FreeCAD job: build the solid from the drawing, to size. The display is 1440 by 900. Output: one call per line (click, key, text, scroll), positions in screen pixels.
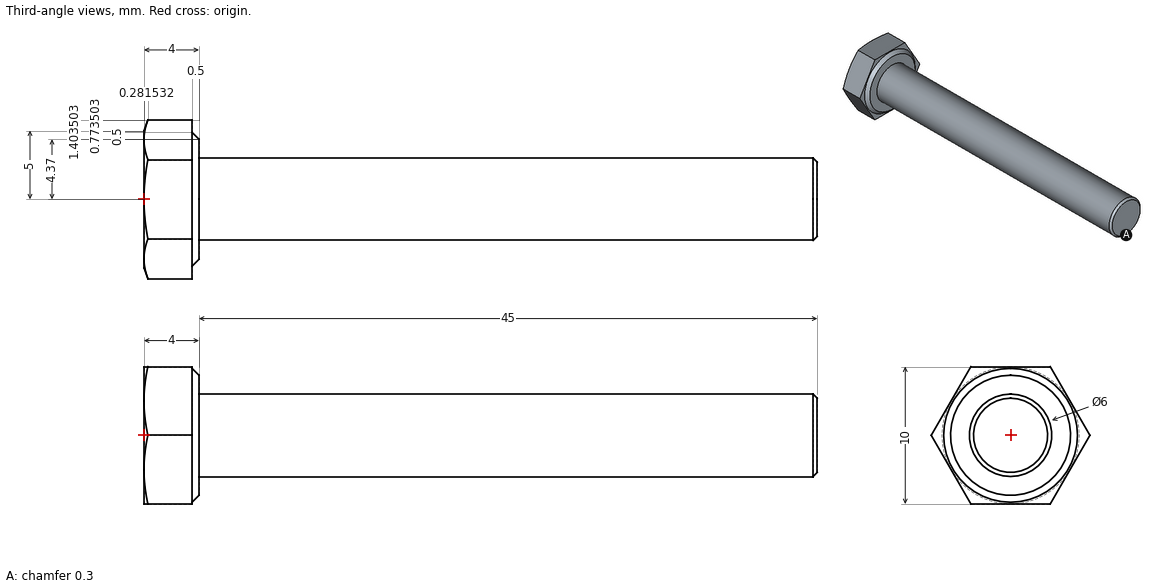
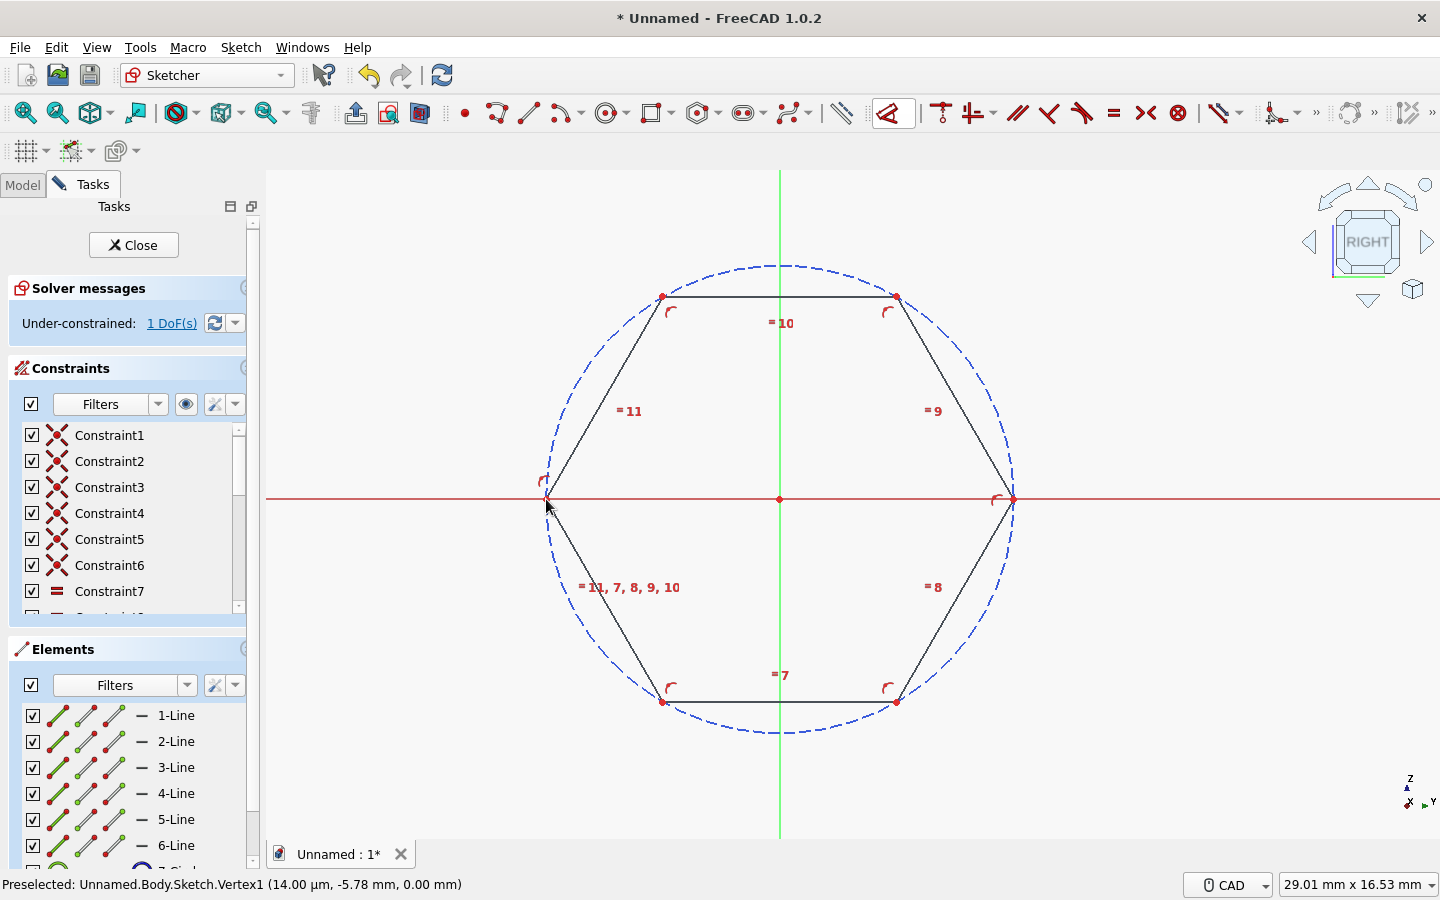
click(888, 114)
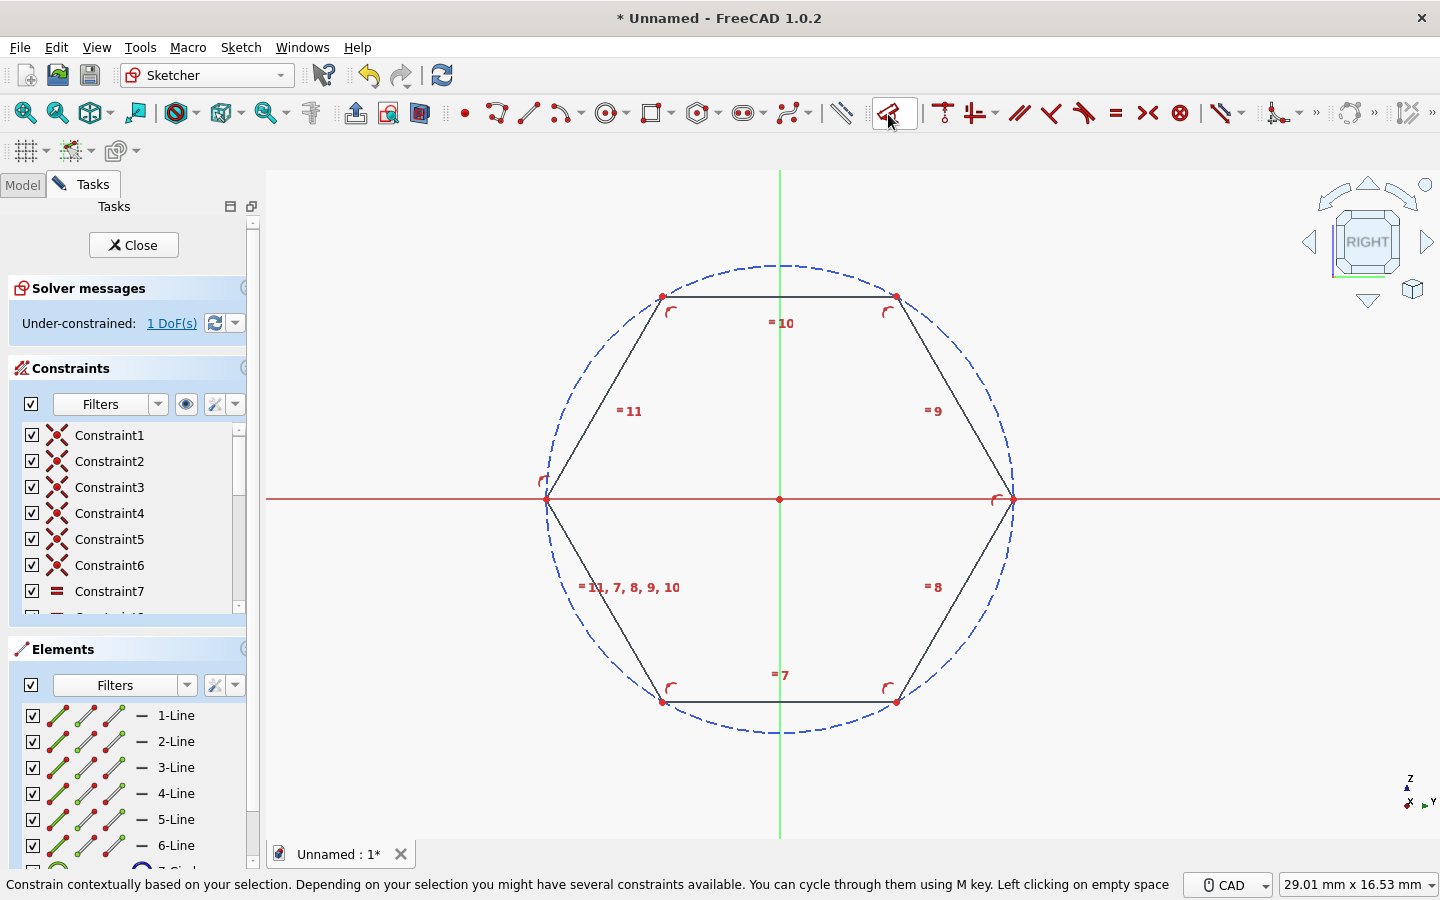
click(663, 702)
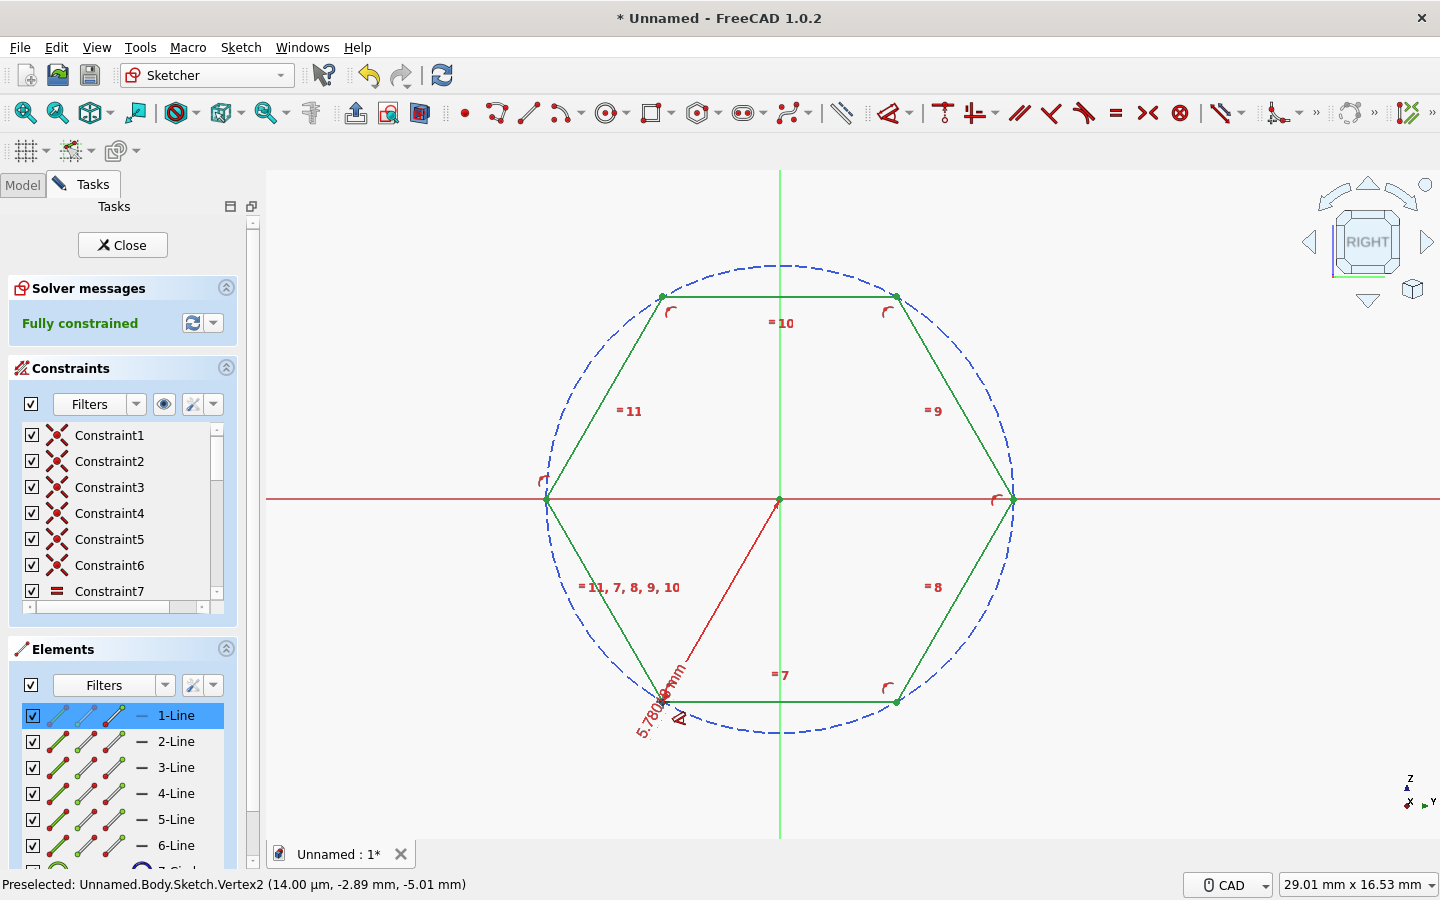
click(897, 297)
click(931, 406)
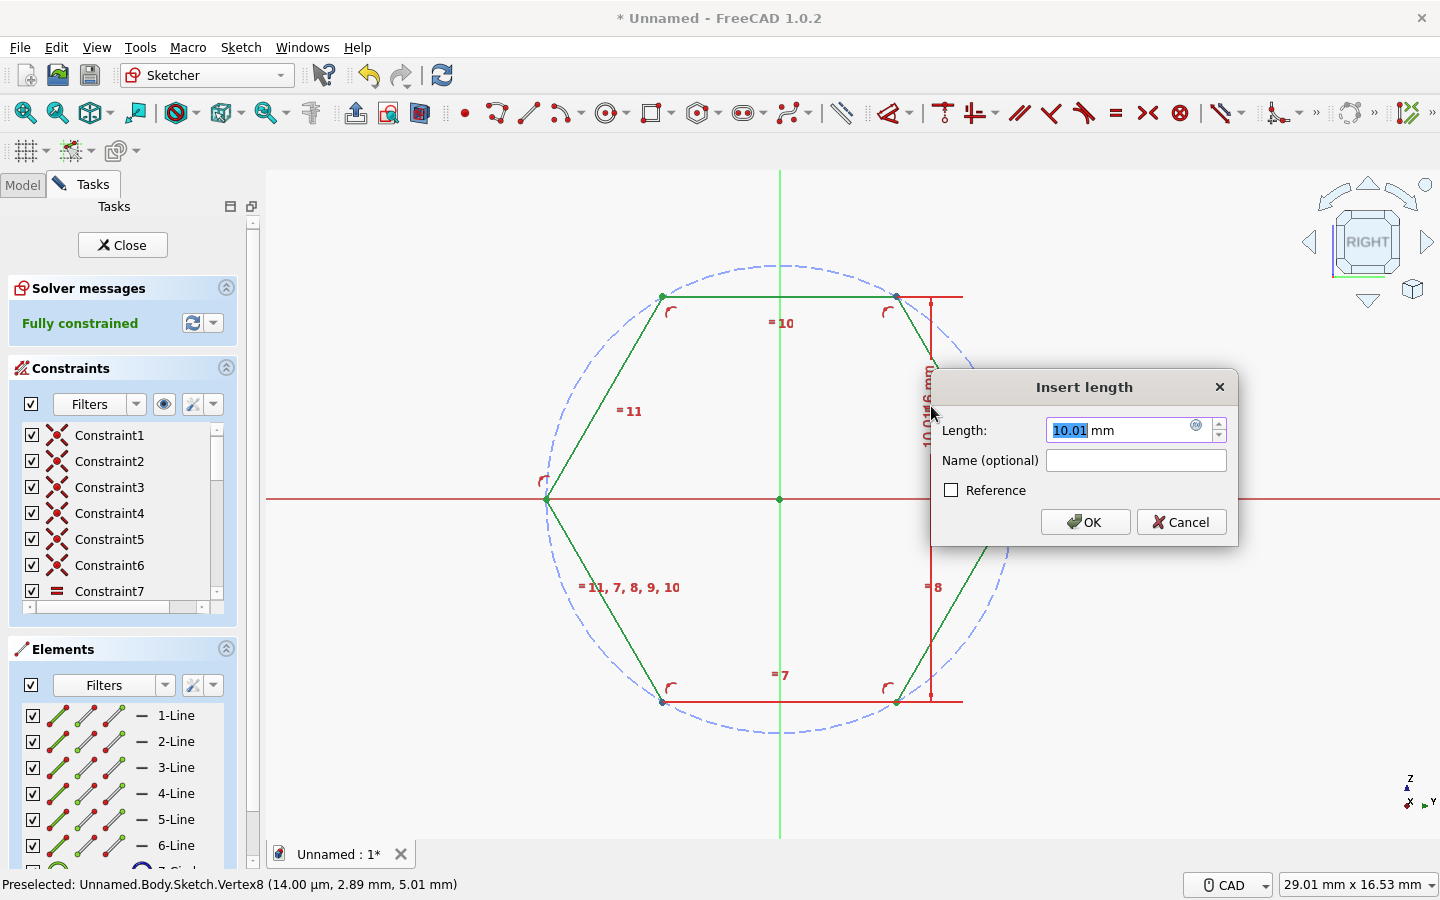
text(10)
key(Return)
key(Escape)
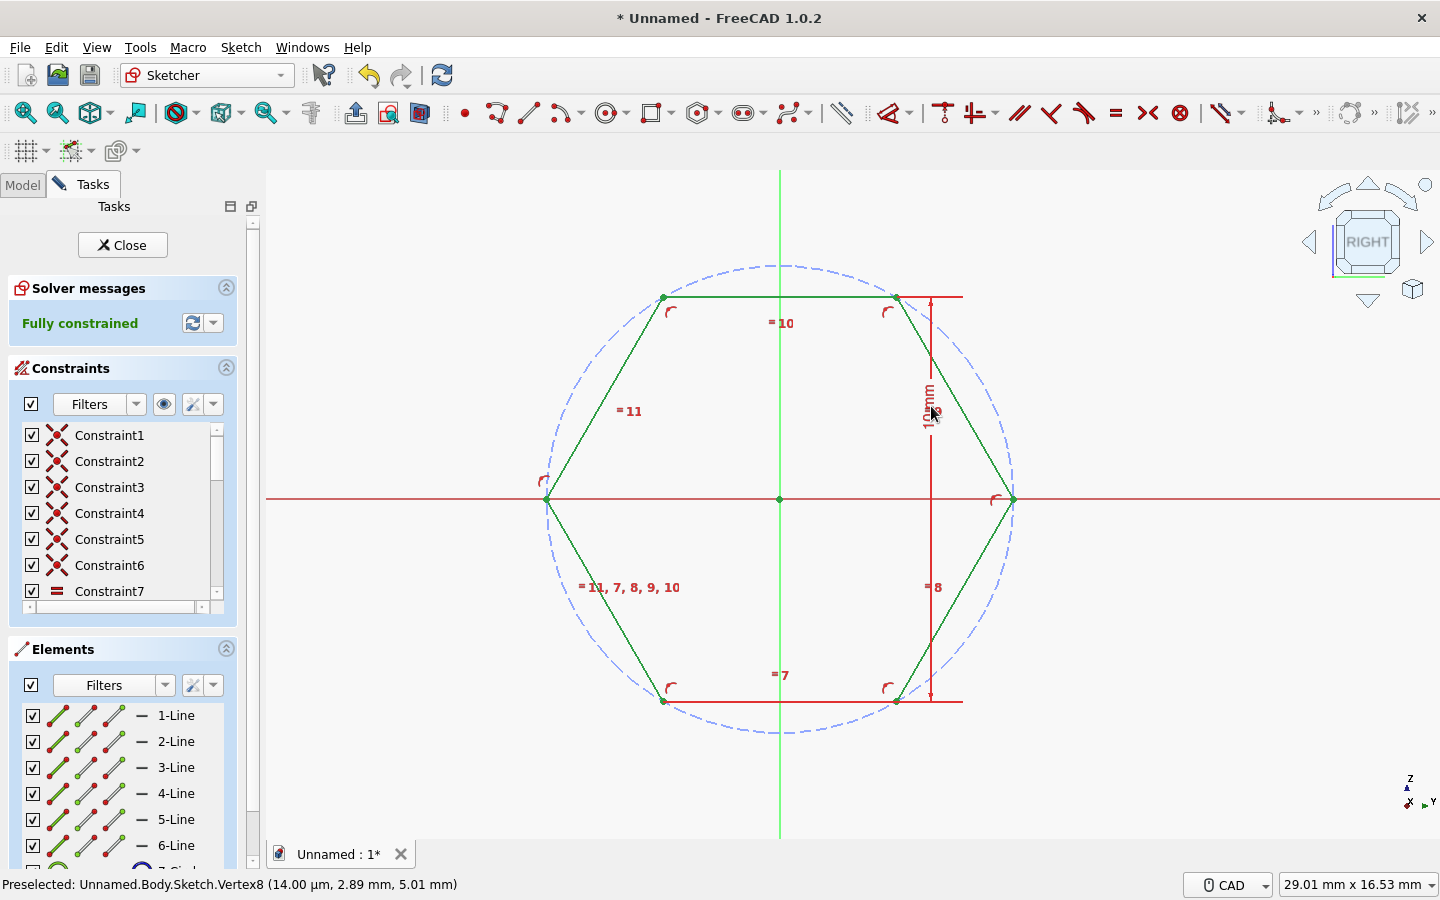
click(123, 245)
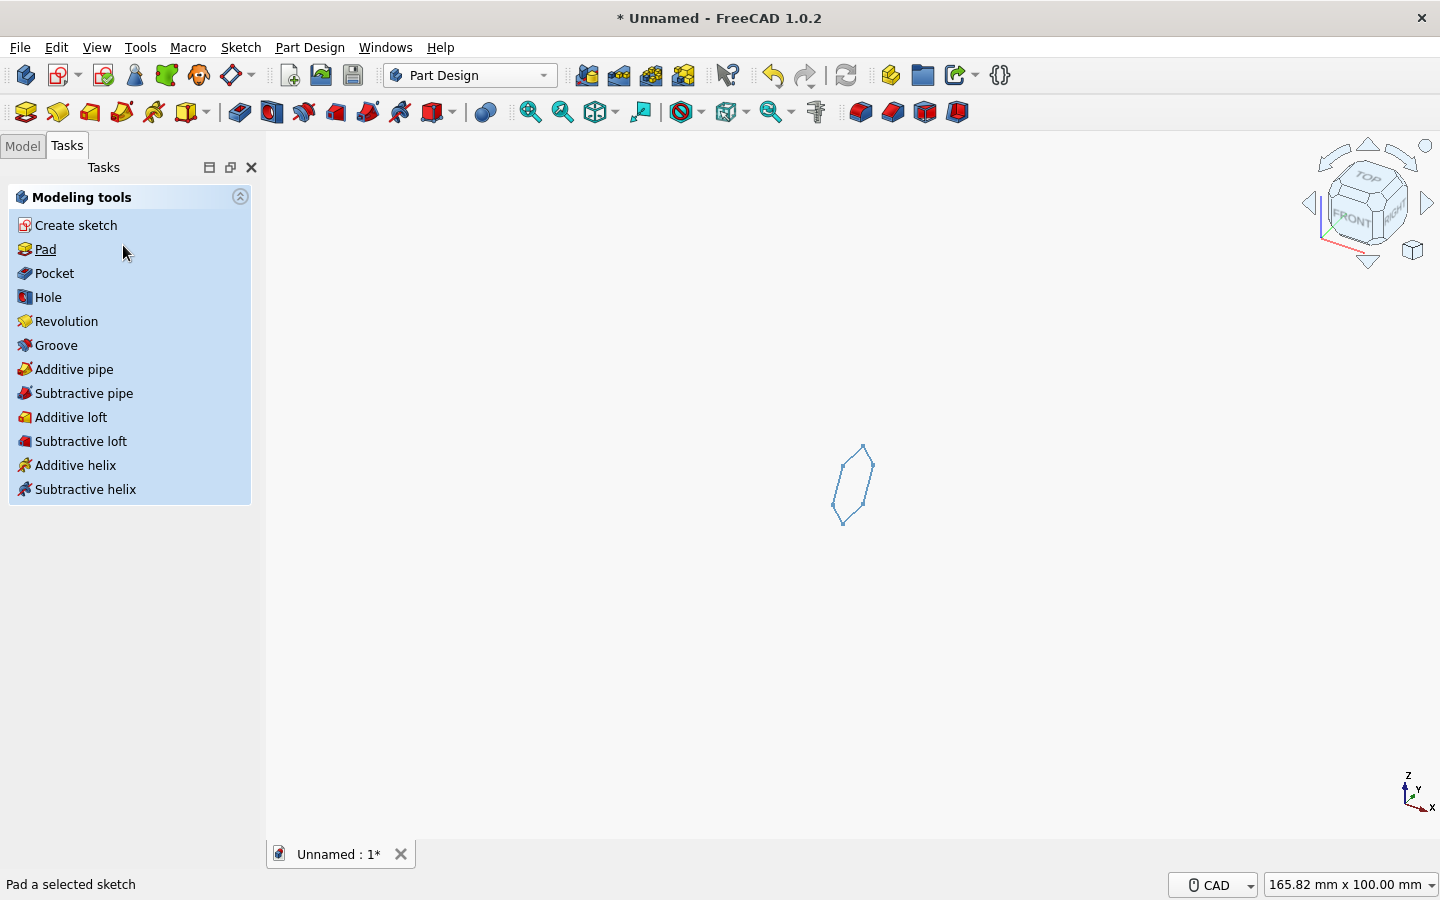
click(26, 112)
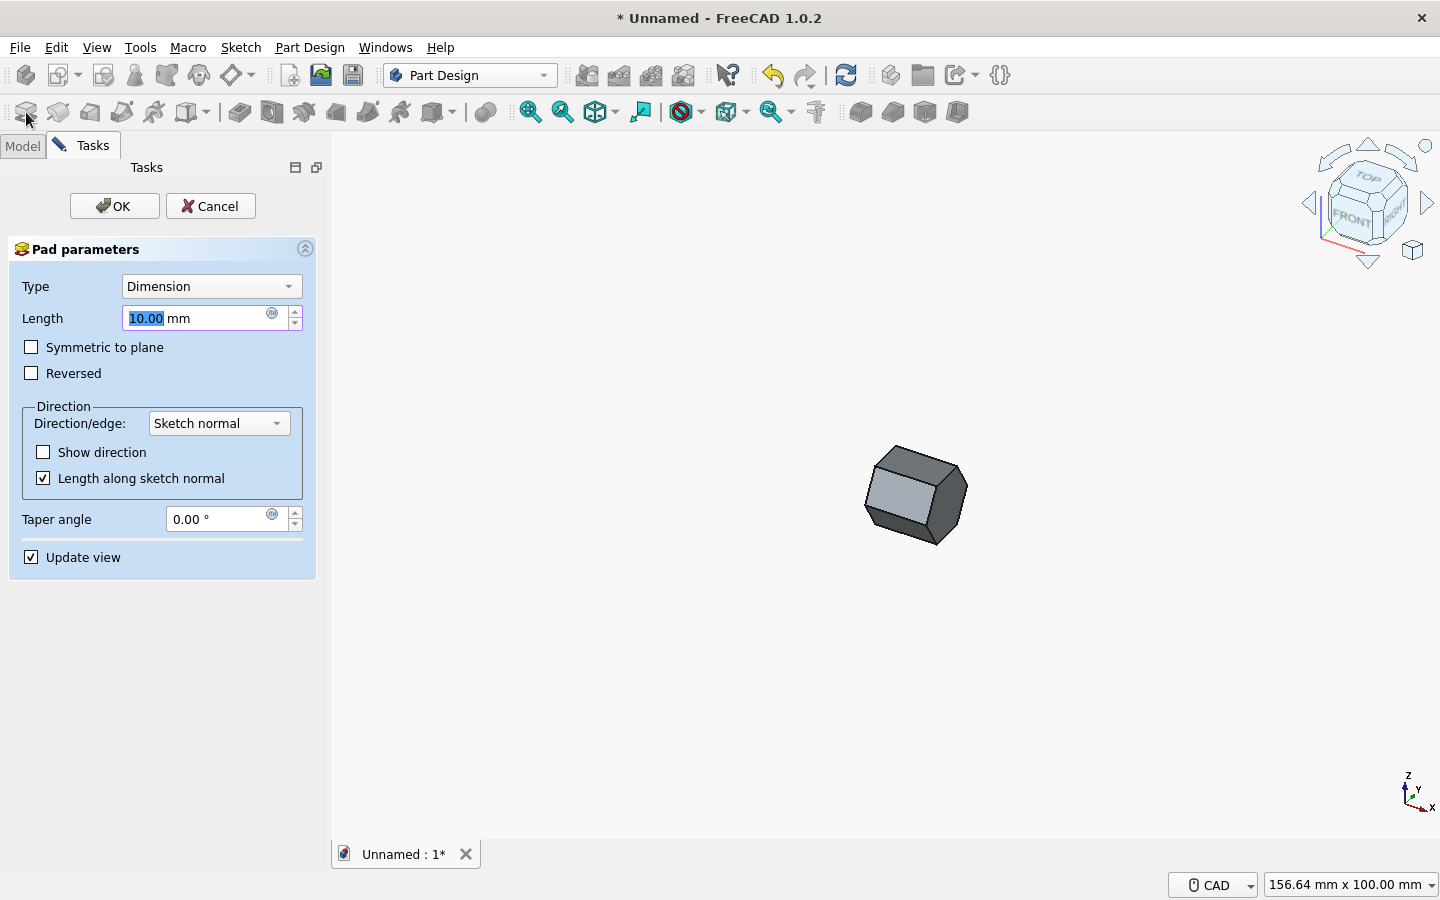
text(4)
key(Tab)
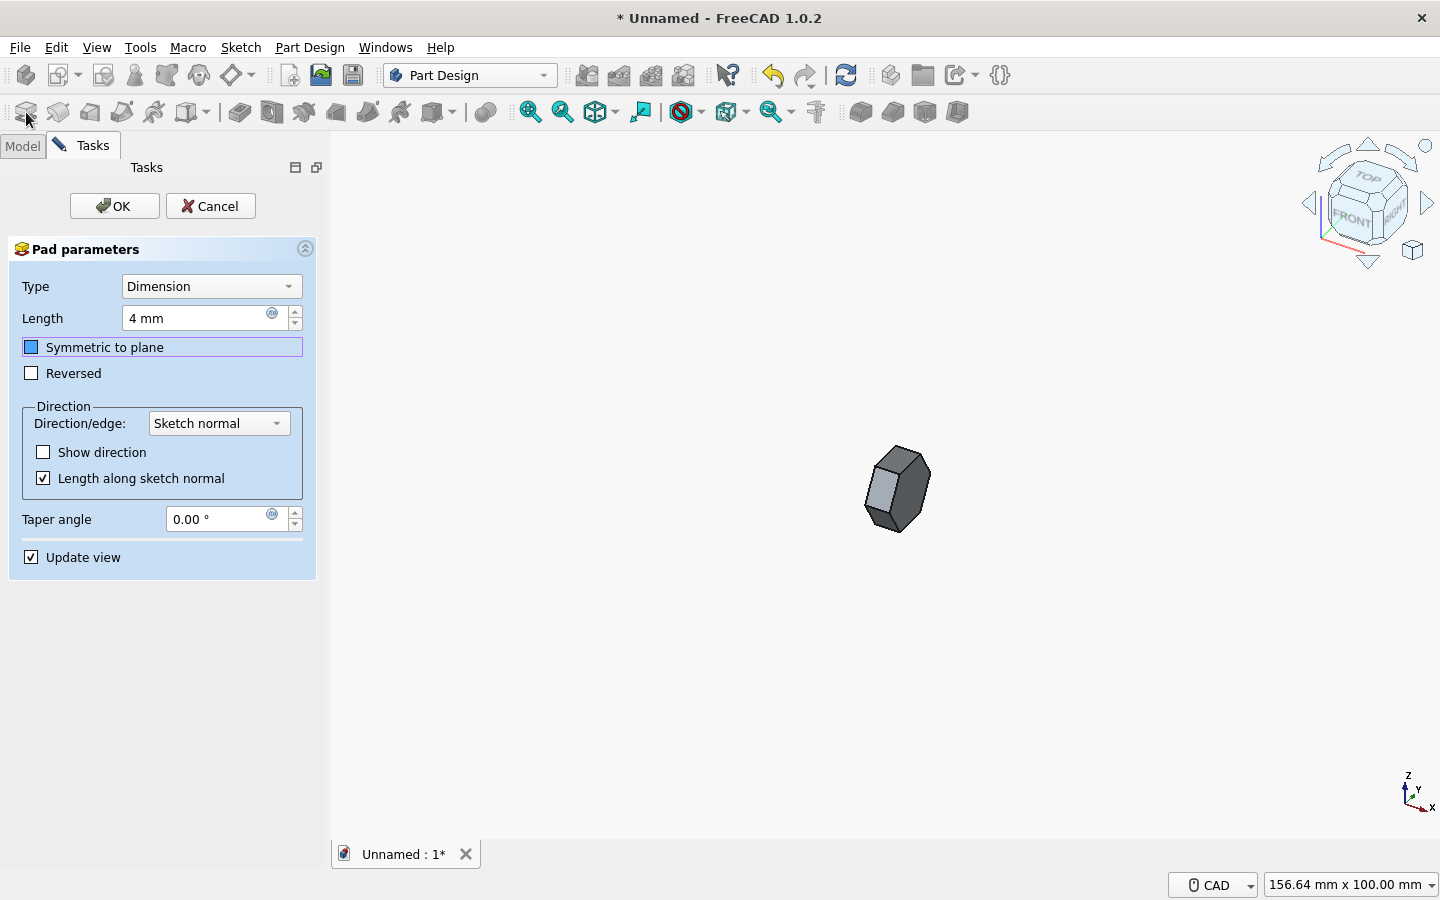
click(115, 206)